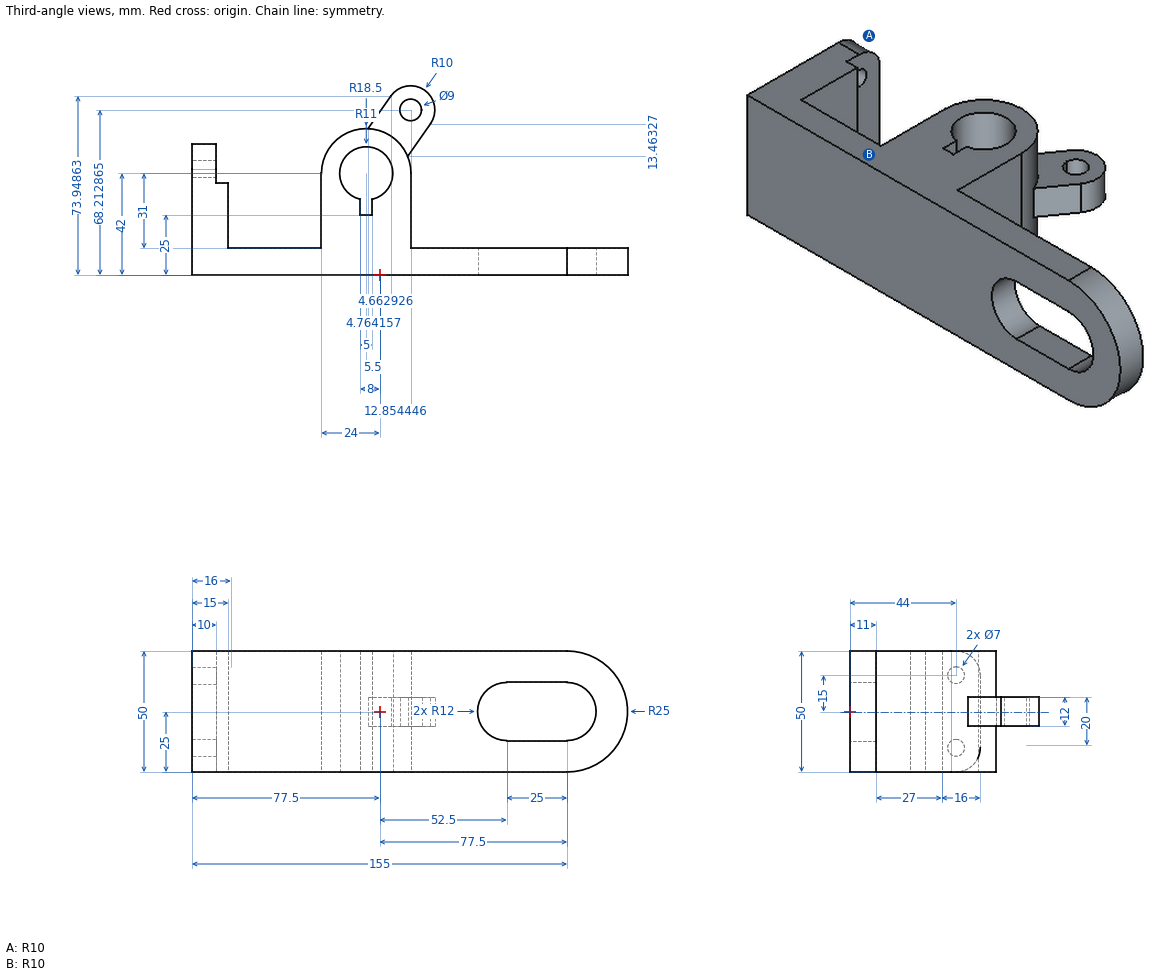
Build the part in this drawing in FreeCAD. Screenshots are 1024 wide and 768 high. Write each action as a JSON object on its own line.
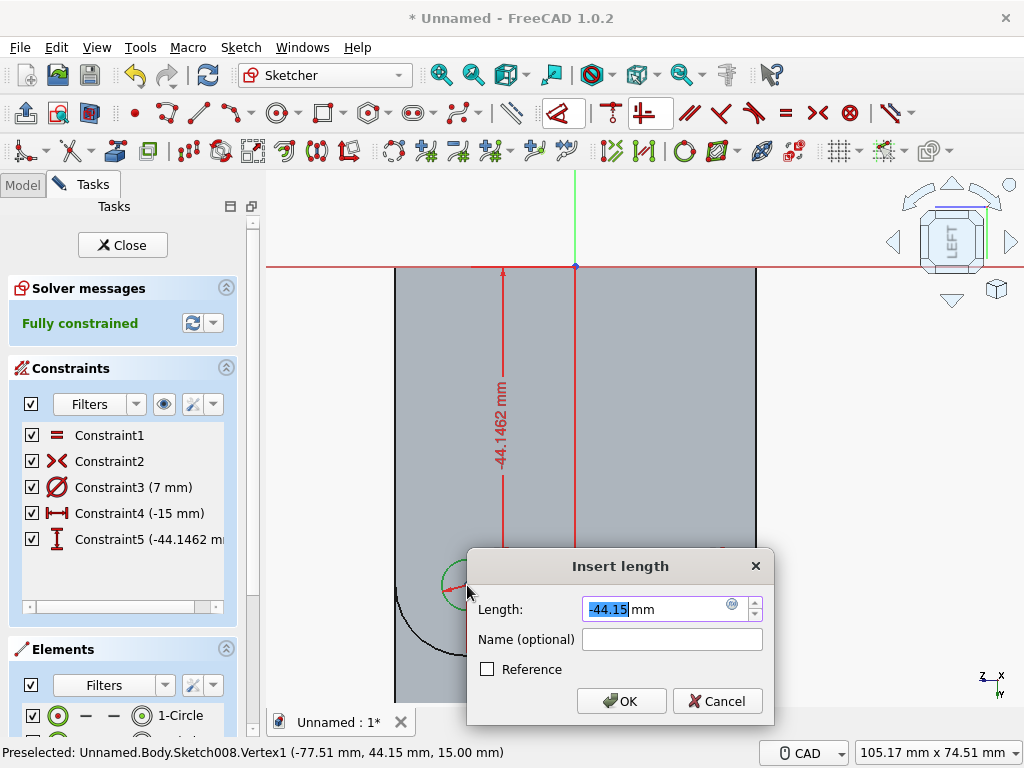
{"action": "type", "text": "-44"}
{"action": "key", "text": "Return"}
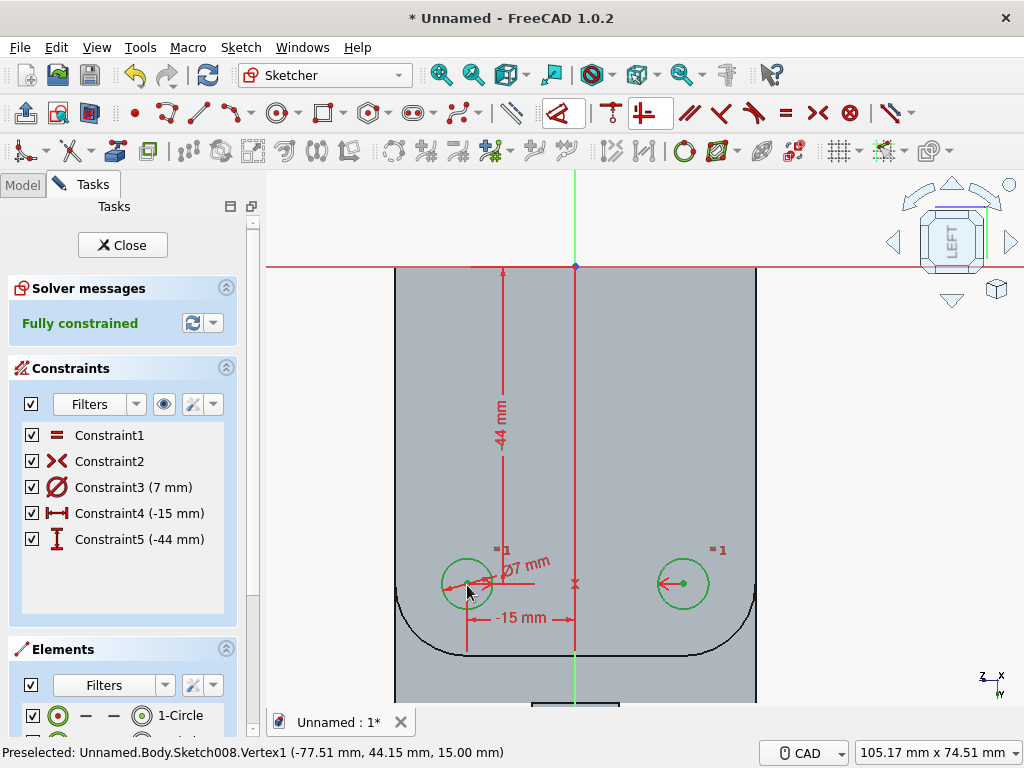
{"action": "left_click", "coordinate": [123, 245]}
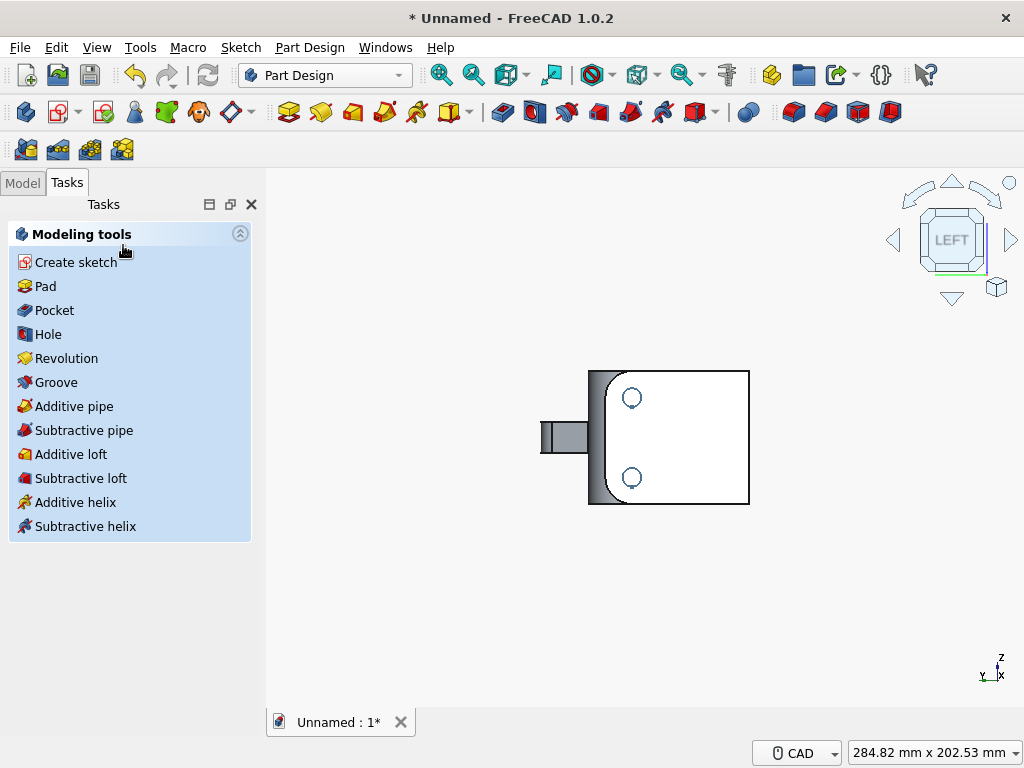
{"action": "left_click", "coordinate": [504, 112]}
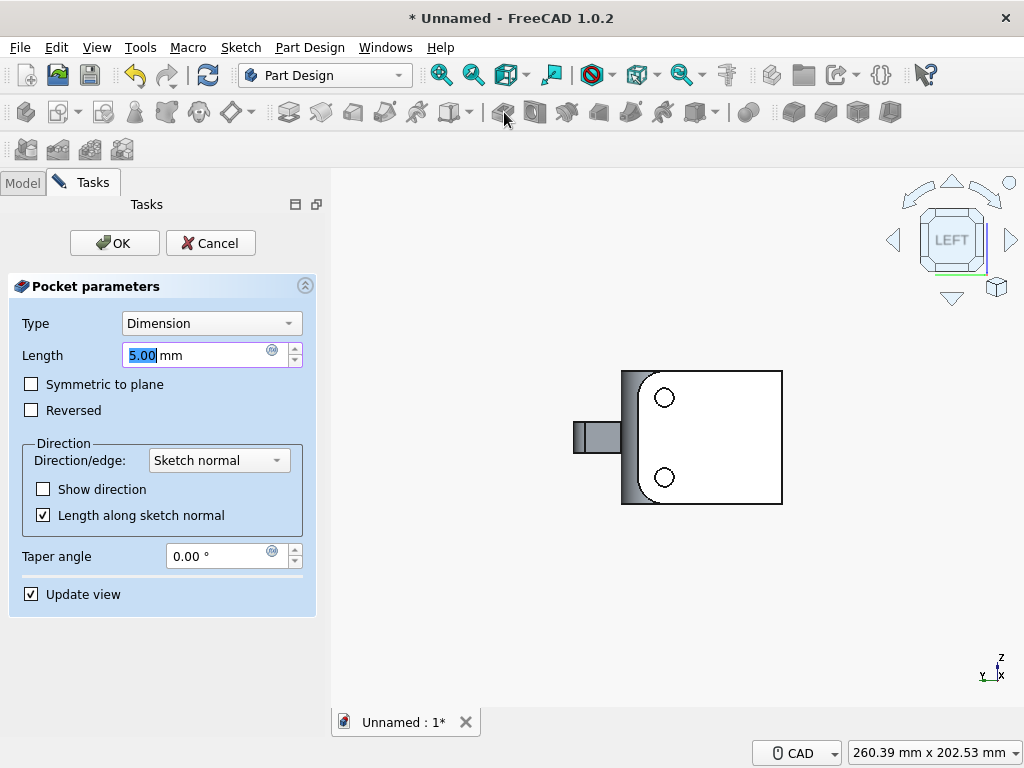
{"action": "type", "text": "16"}
{"action": "key", "text": "Tab"}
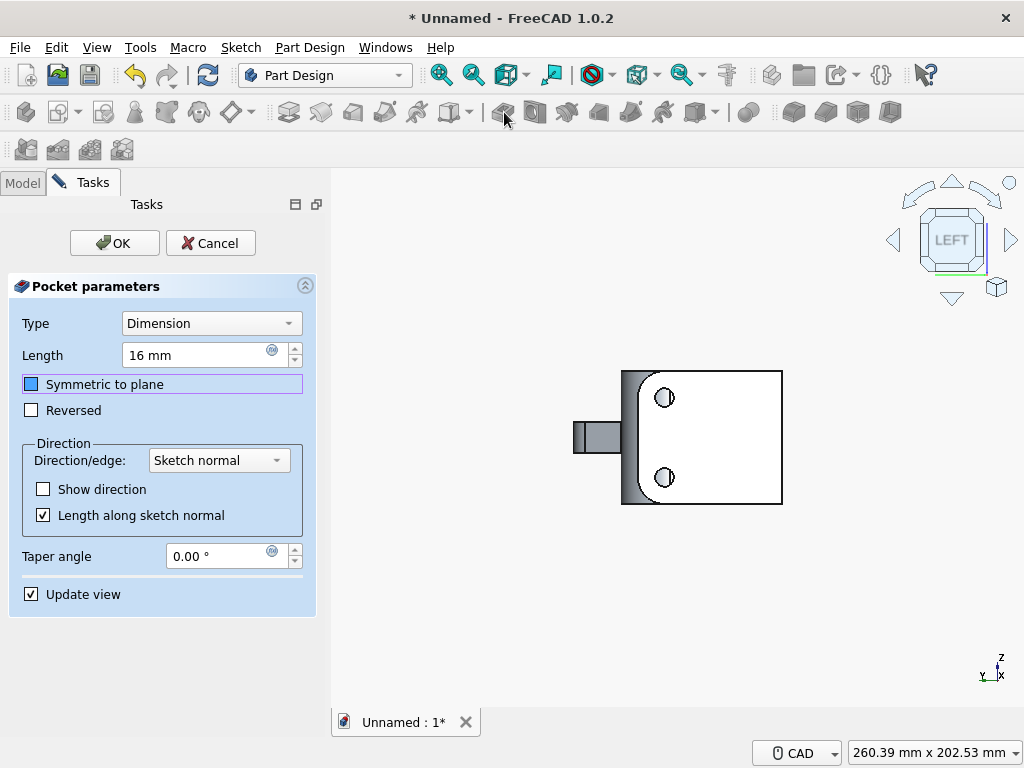
{"action": "left_click", "coordinate": [115, 243]}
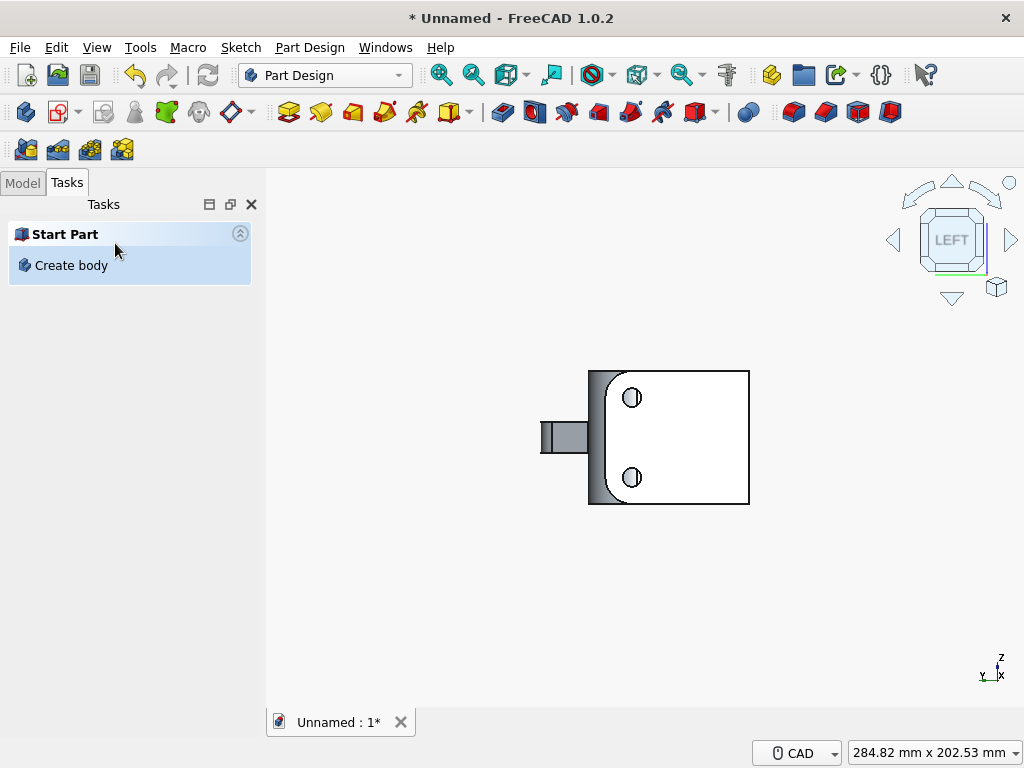
{"action": "key", "text": "0"}